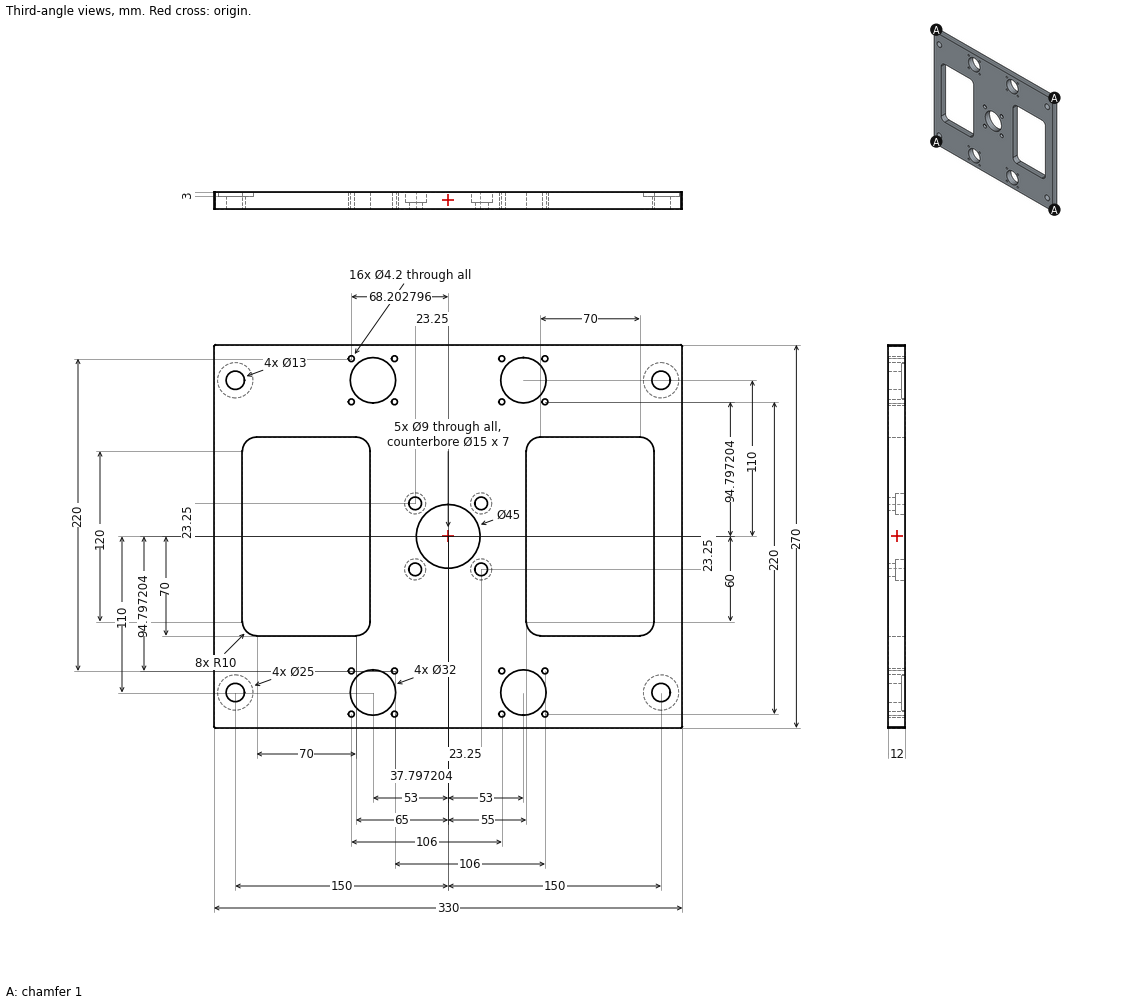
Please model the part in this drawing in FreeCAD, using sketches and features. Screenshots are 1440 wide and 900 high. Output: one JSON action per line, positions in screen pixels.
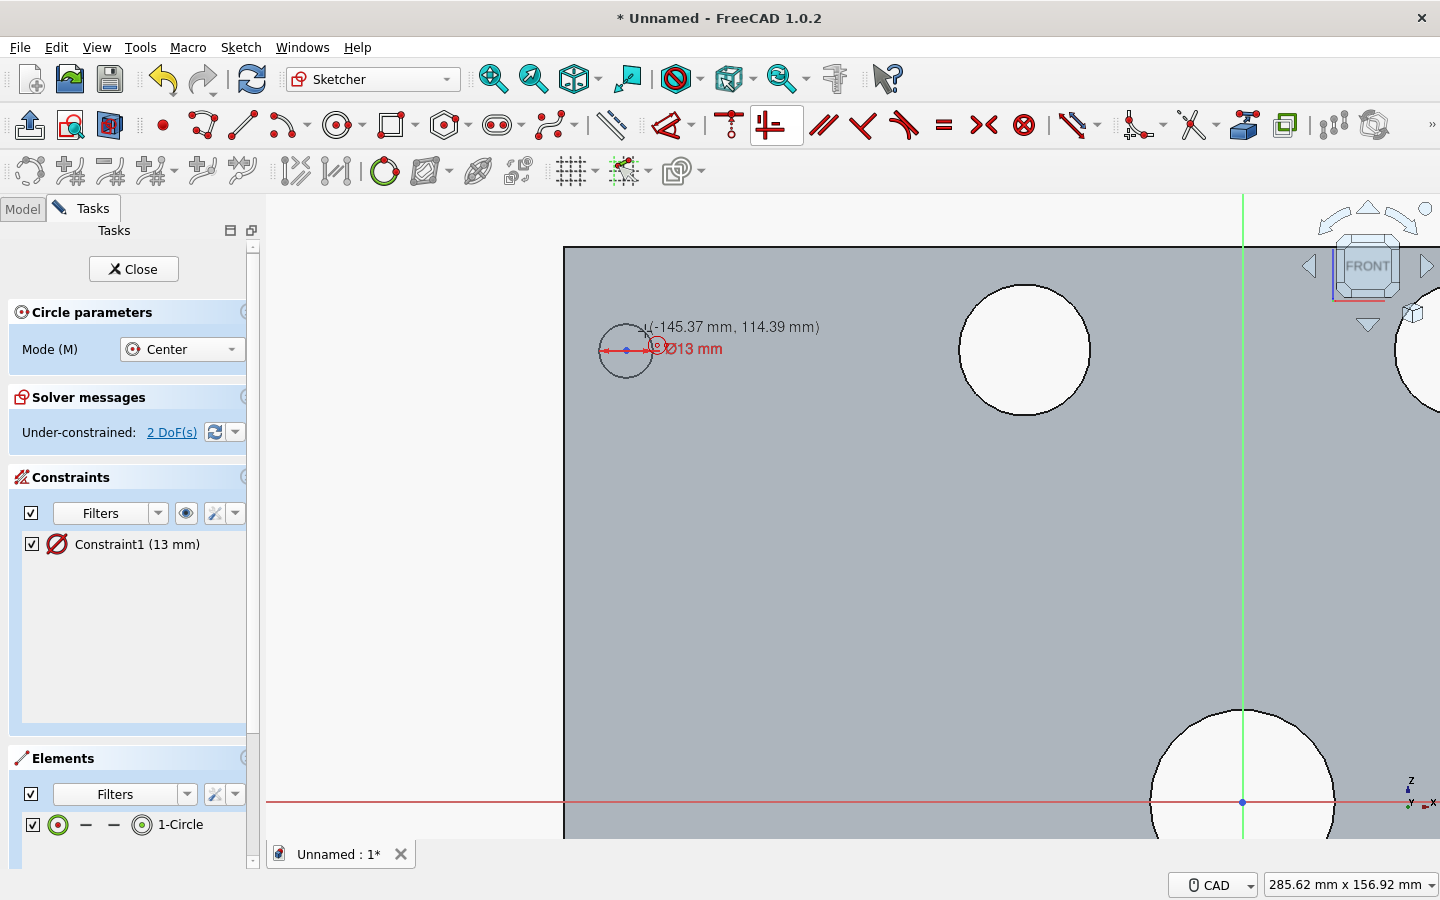
{"action": "scroll", "coordinate": [411, 283], "scroll_direction": "down", "scroll_amount": 4}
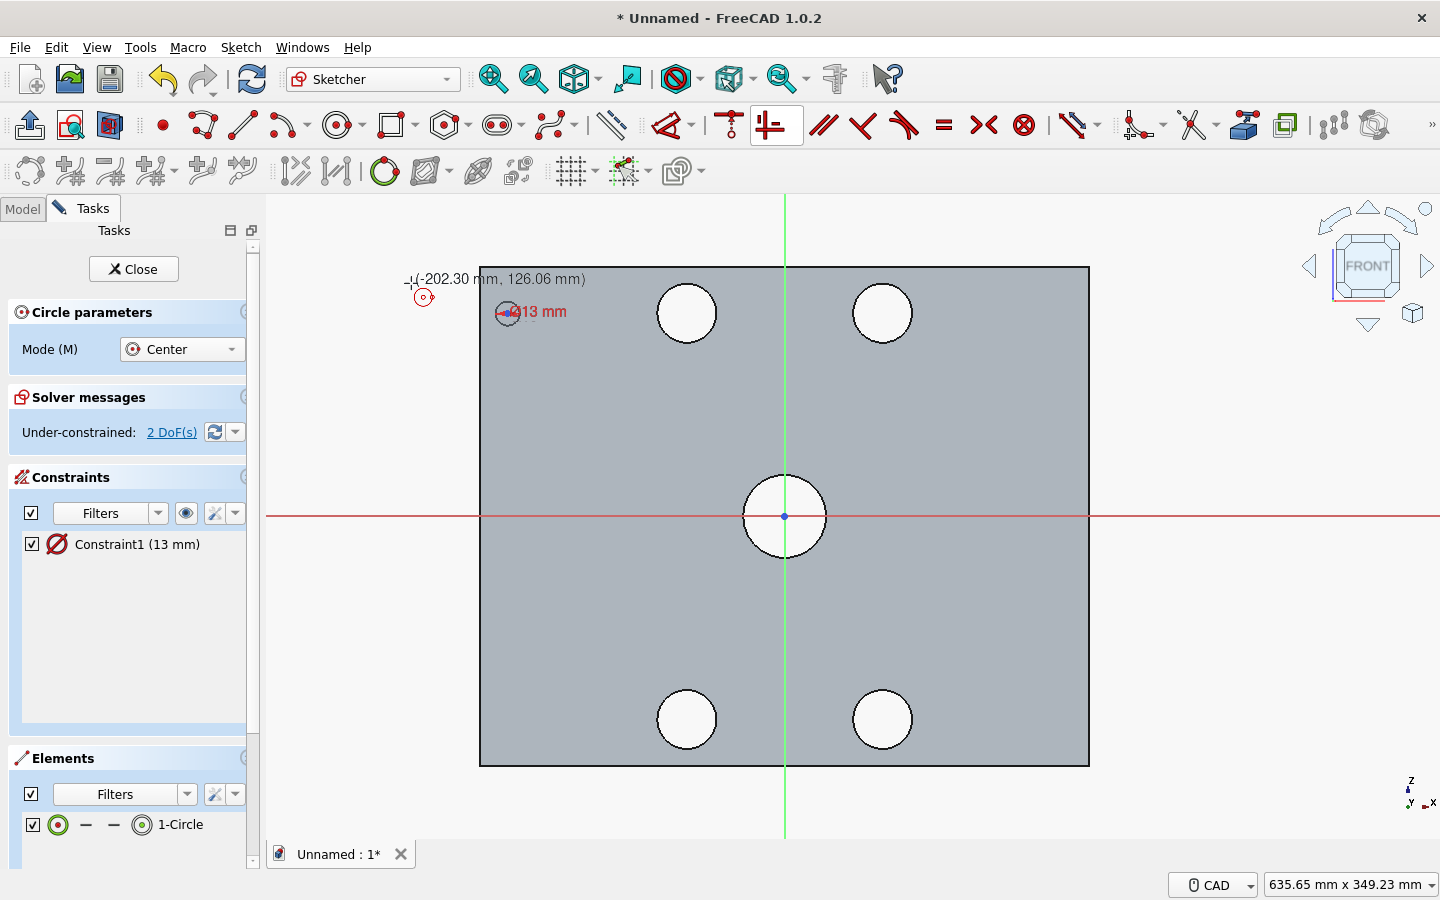
{"action": "scroll", "coordinate": [1062, 313], "scroll_direction": "up", "scroll_amount": 4}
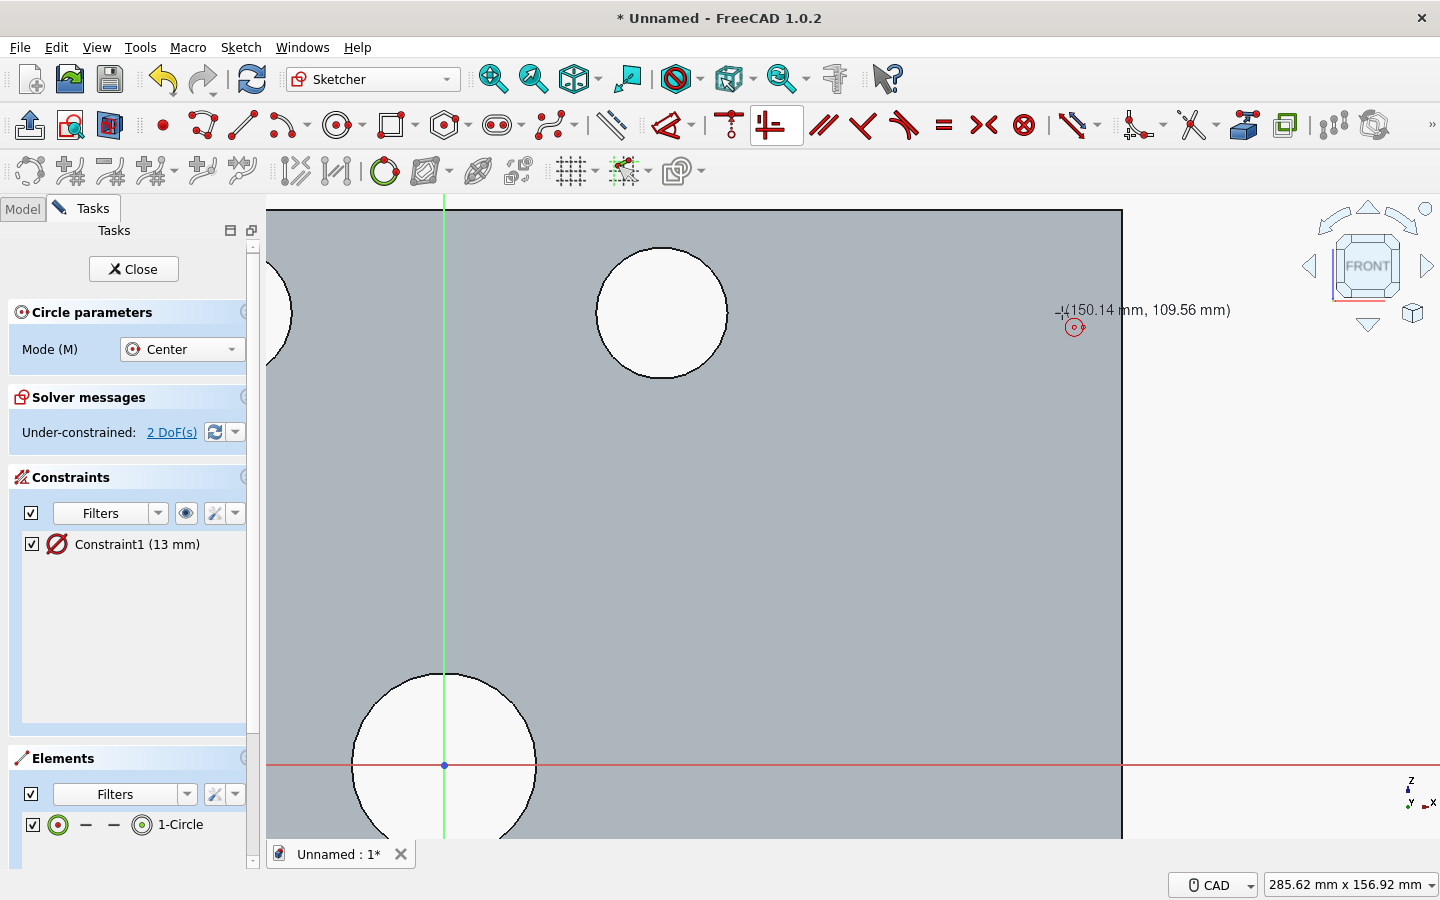
{"action": "left_click", "coordinate": [1061, 313]}
{"action": "mouse_move", "coordinate": [1079, 294]}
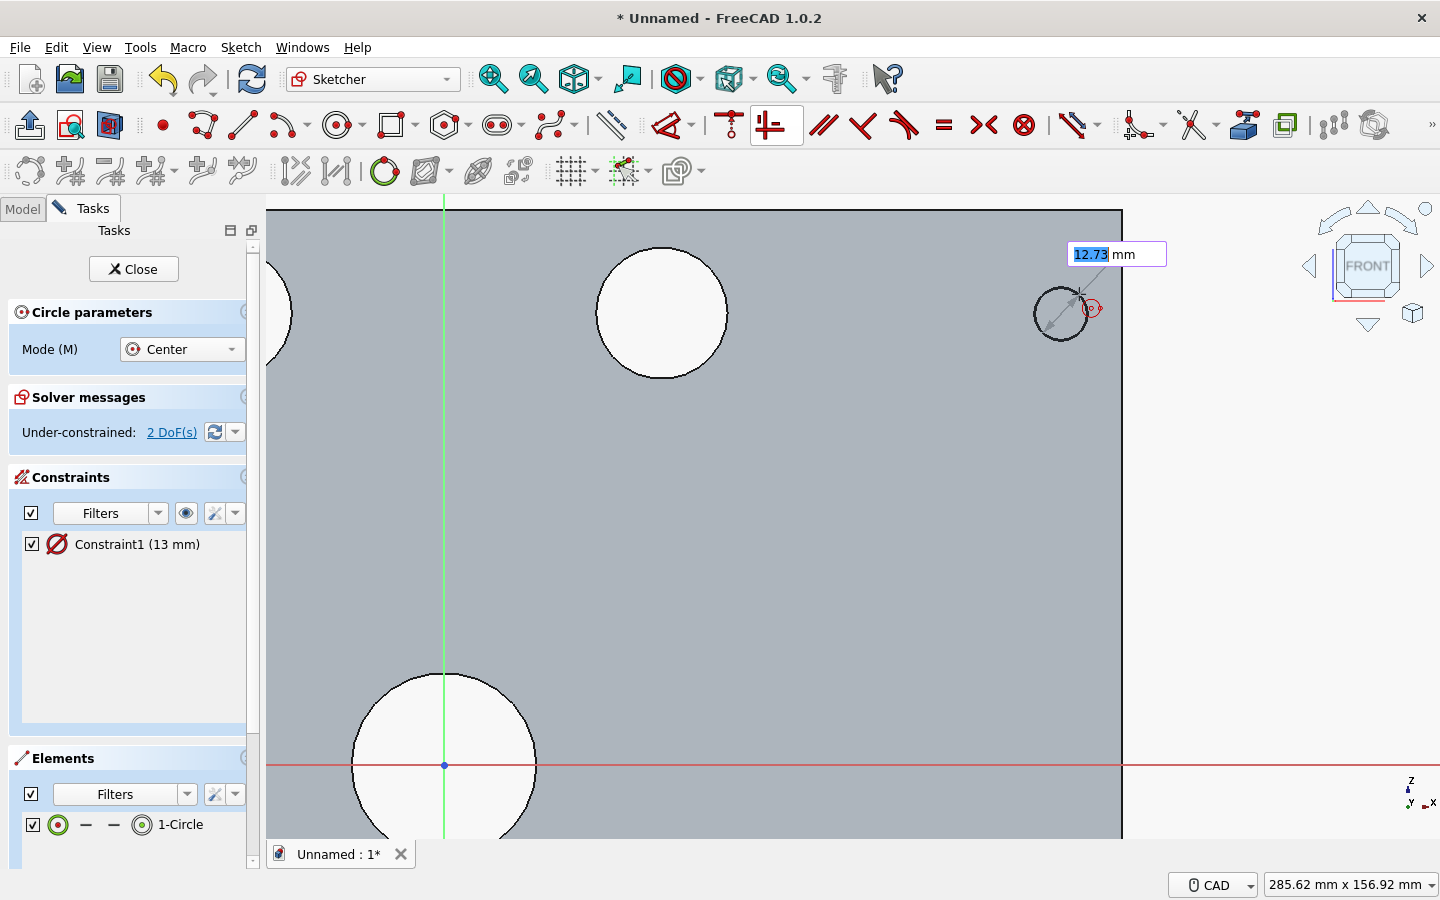
{"action": "type", "text": "13"}
{"action": "key", "text": "Return"}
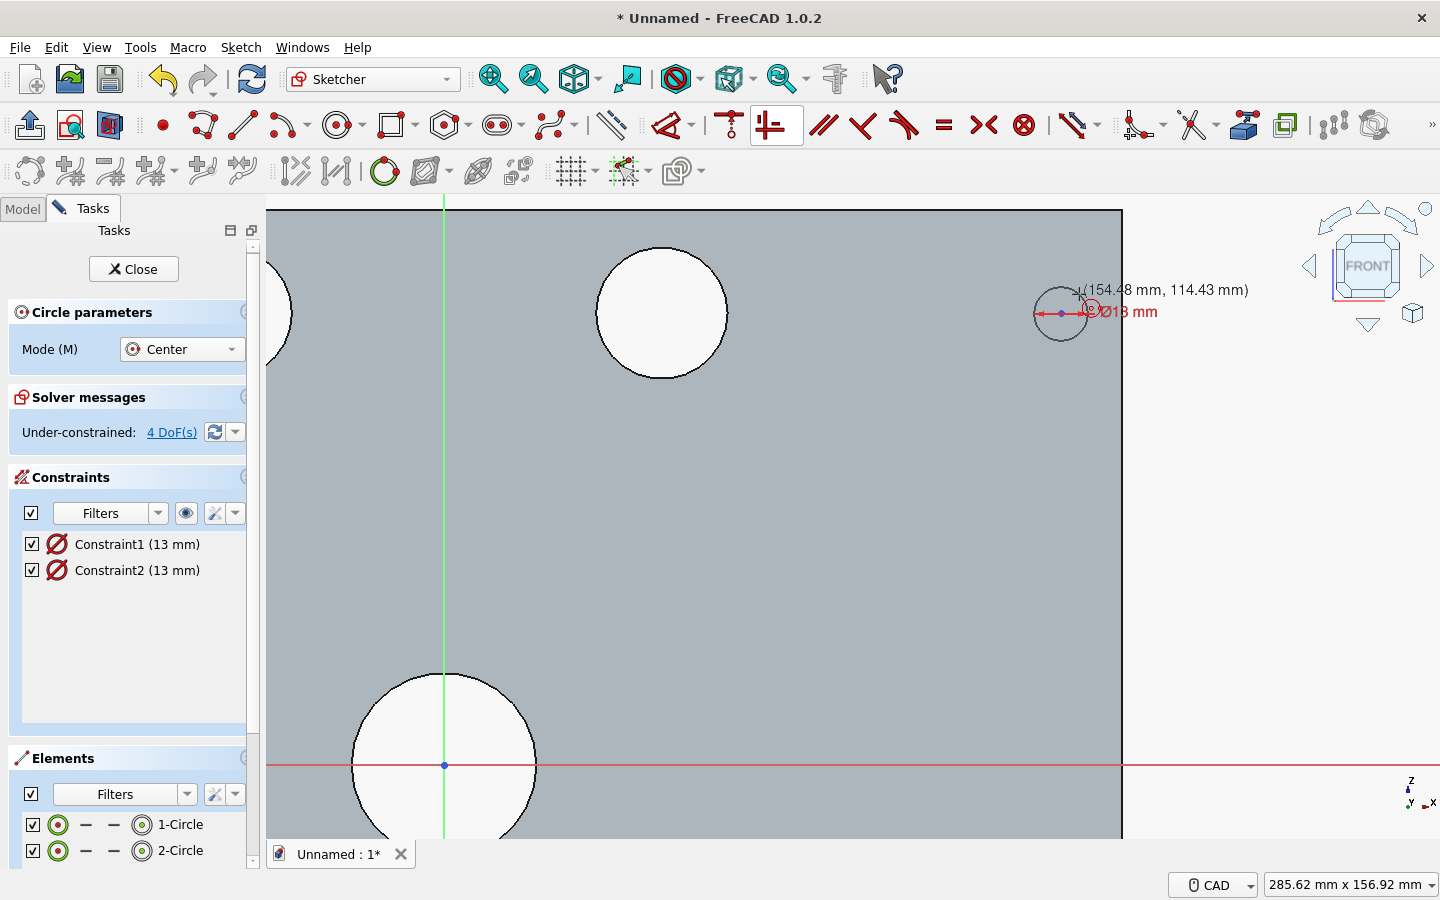
{"action": "scroll", "coordinate": [1062, 313], "scroll_direction": "down", "scroll_amount": 4}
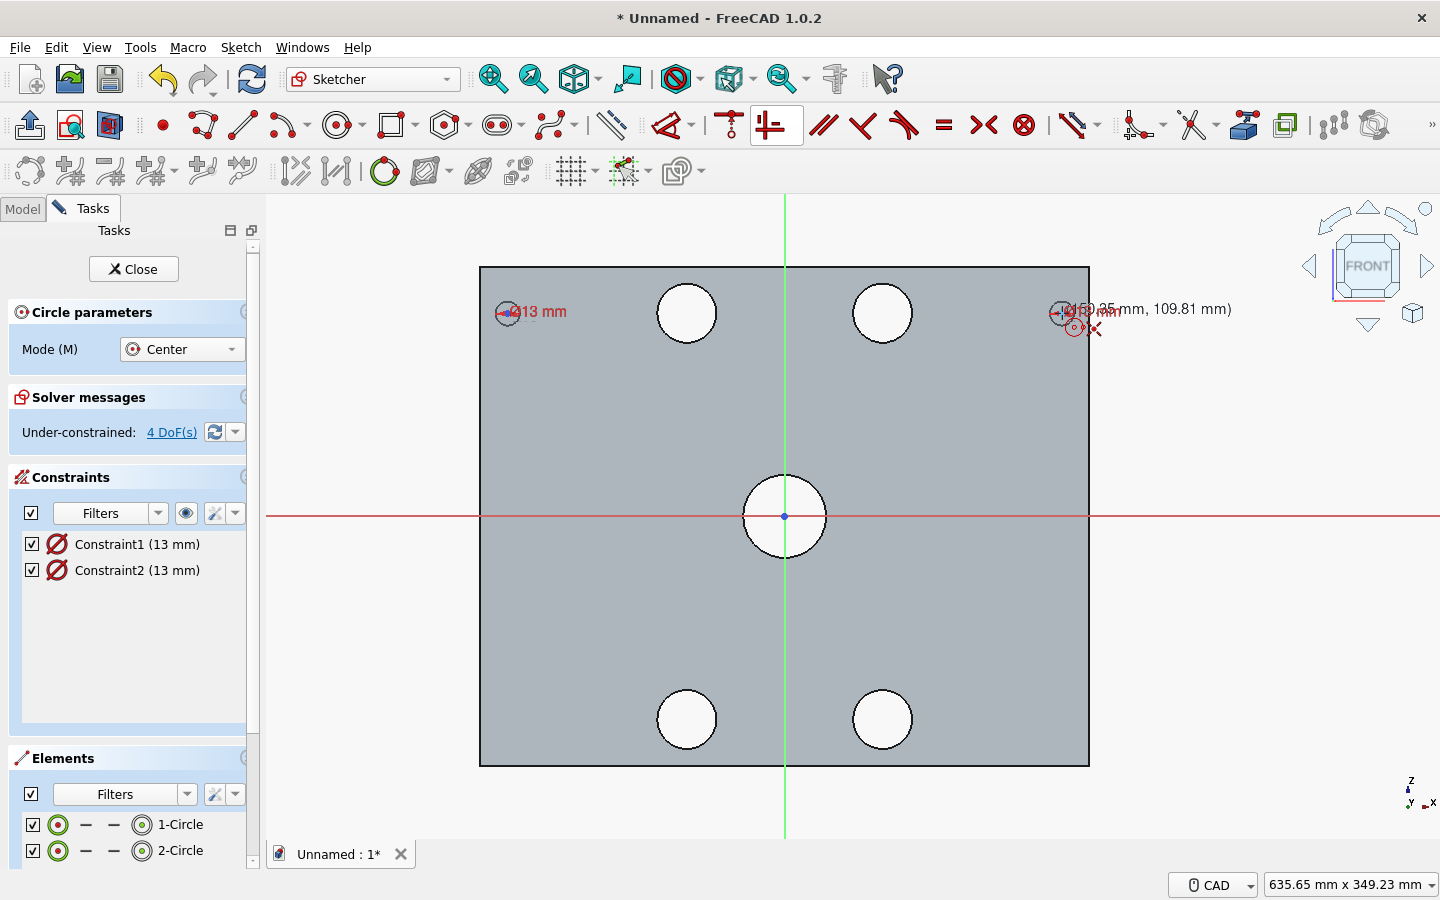
{"action": "scroll", "coordinate": [508, 720], "scroll_direction": "up", "scroll_amount": 4}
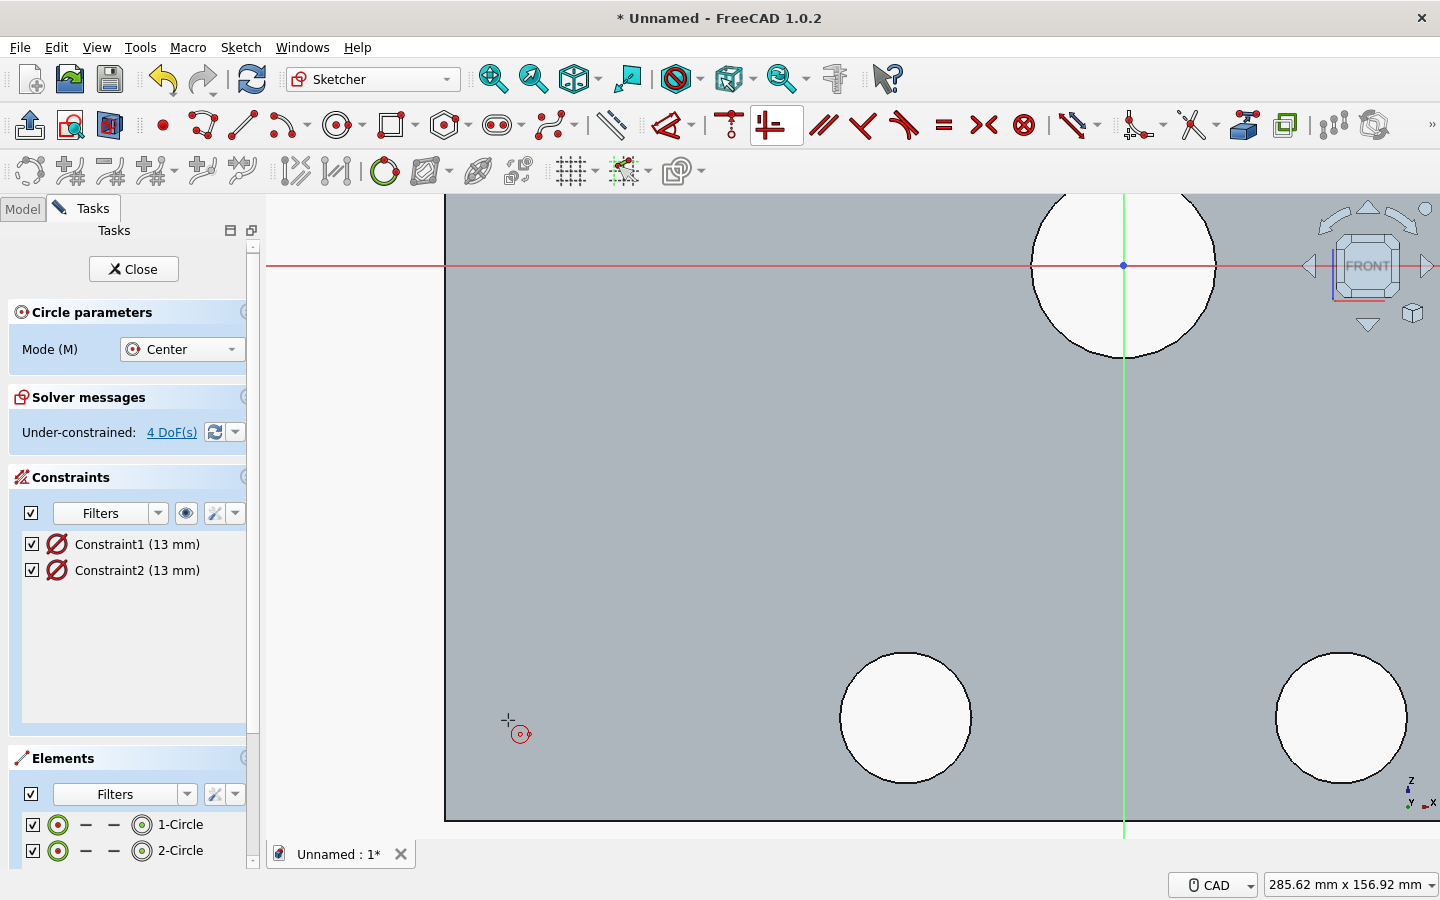
{"action": "left_click", "coordinate": [507, 718]}
{"action": "mouse_move", "coordinate": [526, 699]}